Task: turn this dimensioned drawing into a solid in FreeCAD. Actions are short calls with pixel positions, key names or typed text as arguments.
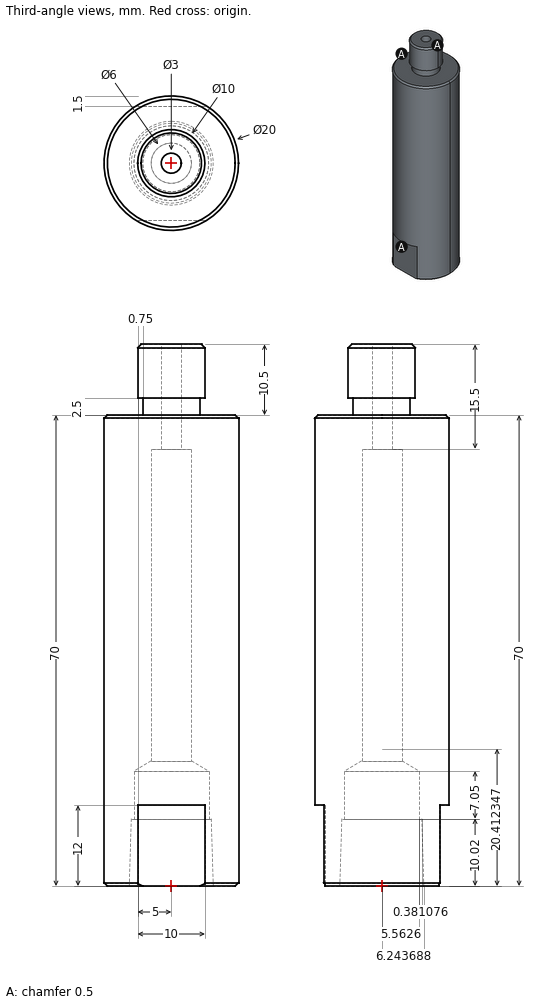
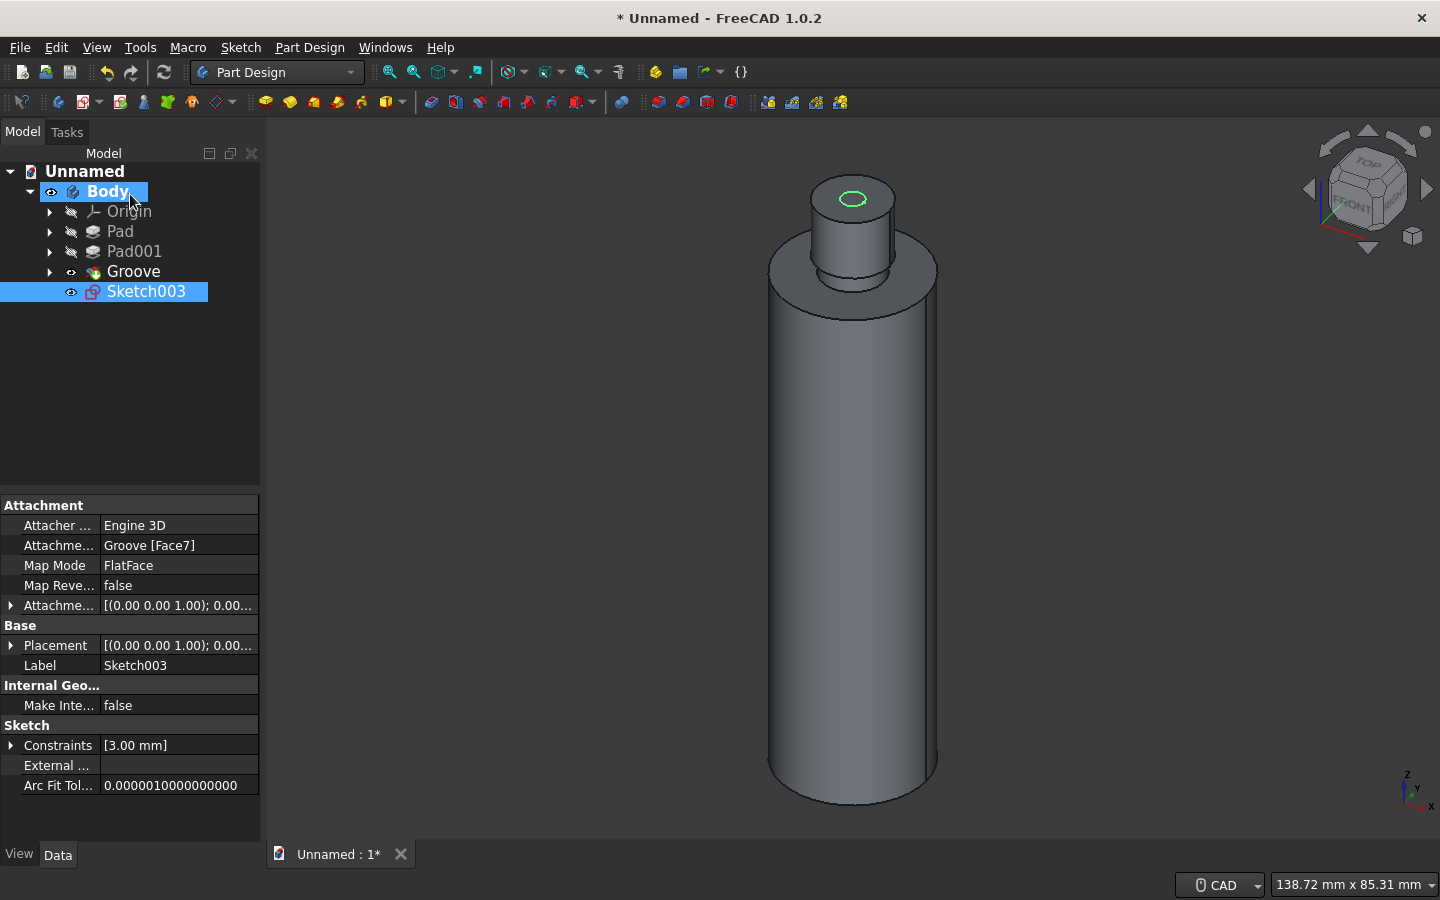
click(432, 102)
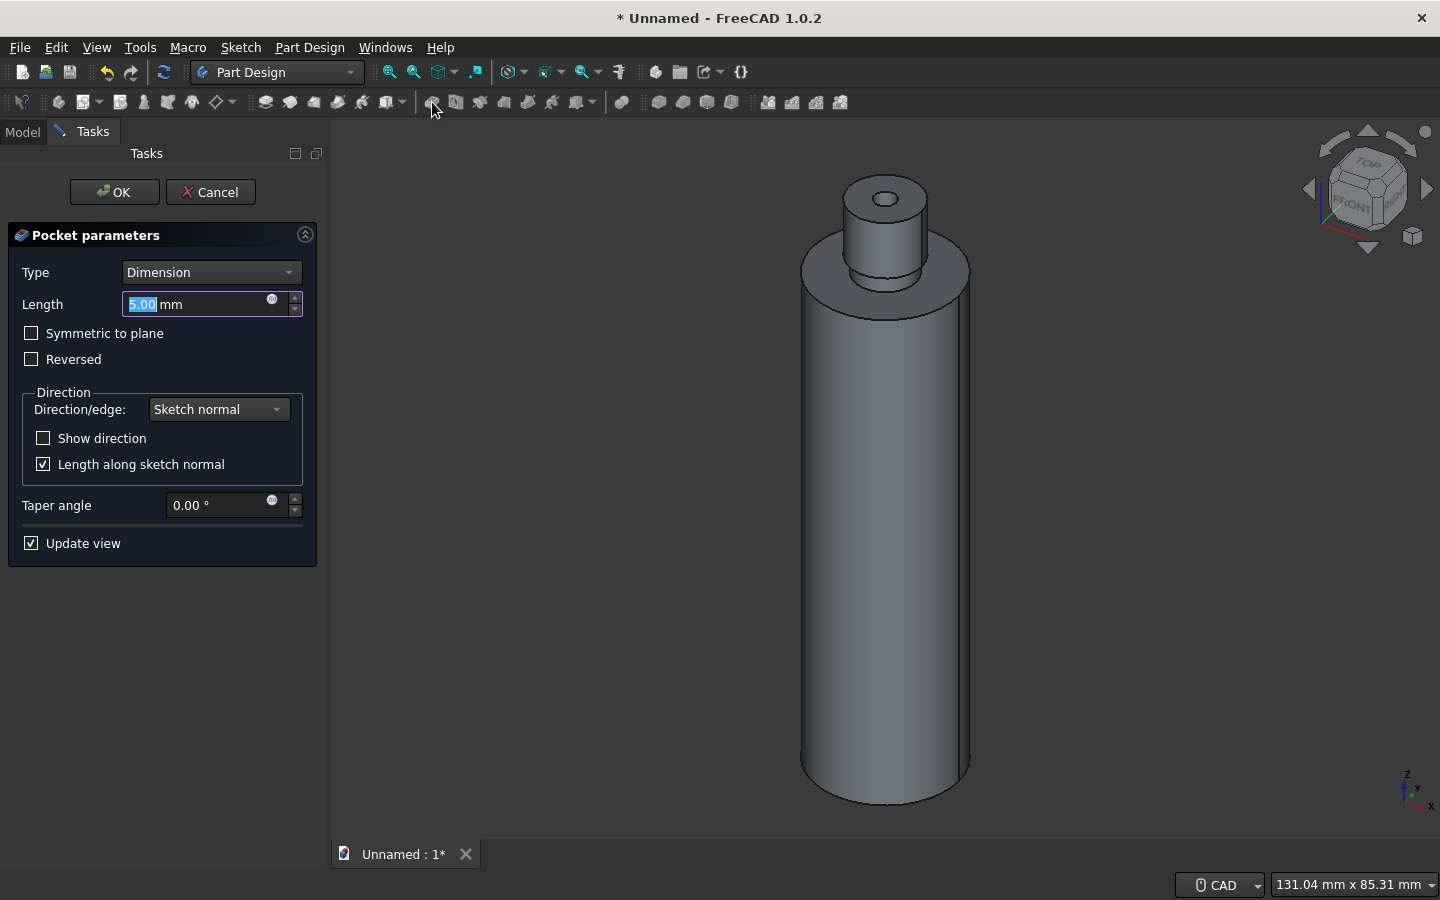
text(15.5)
key(Tab)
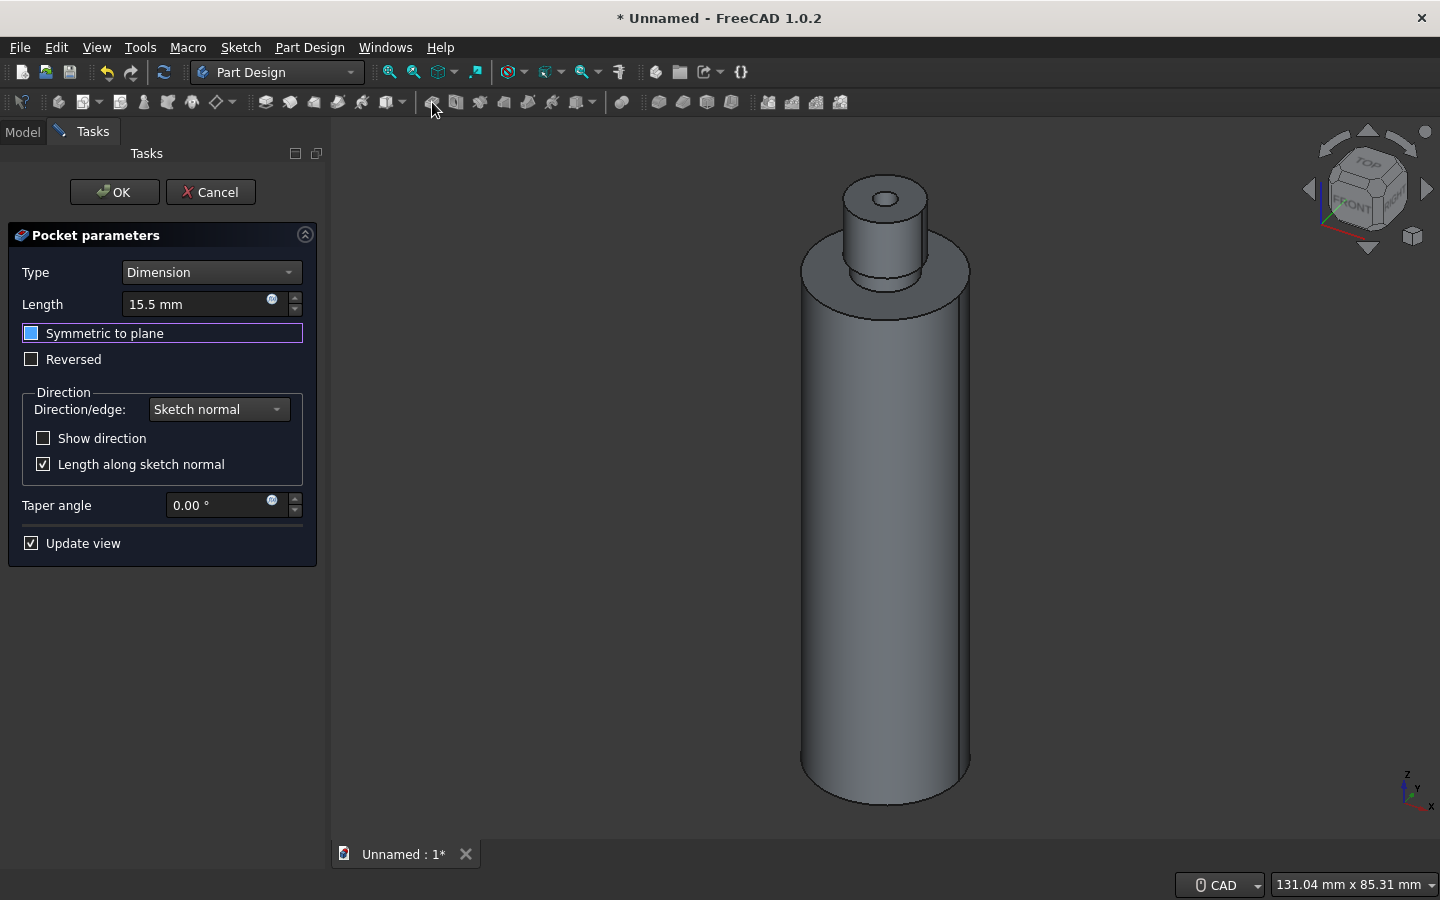
click(115, 192)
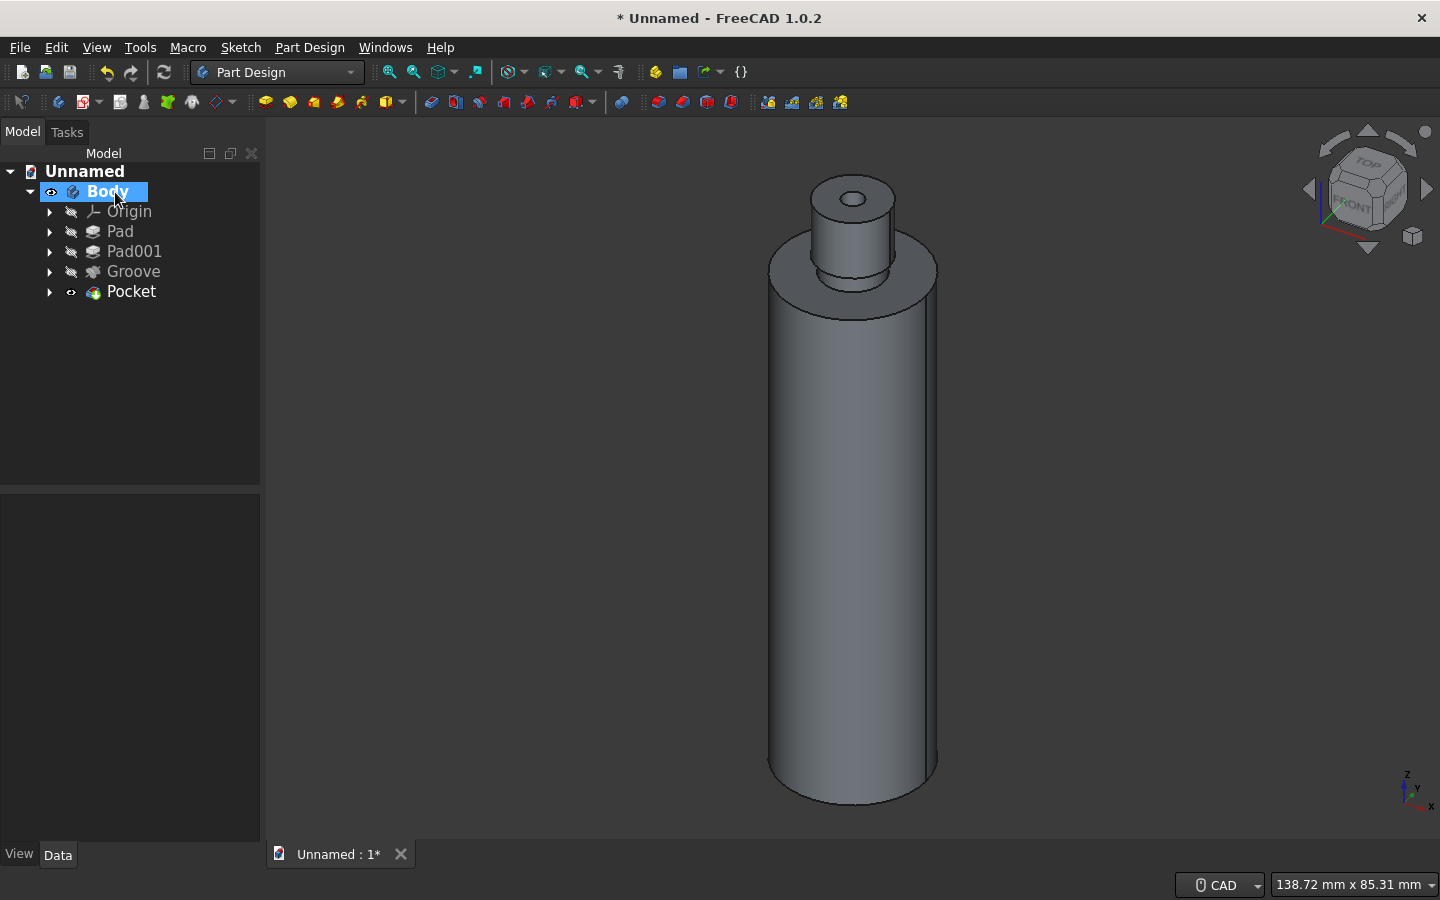
click(84, 102)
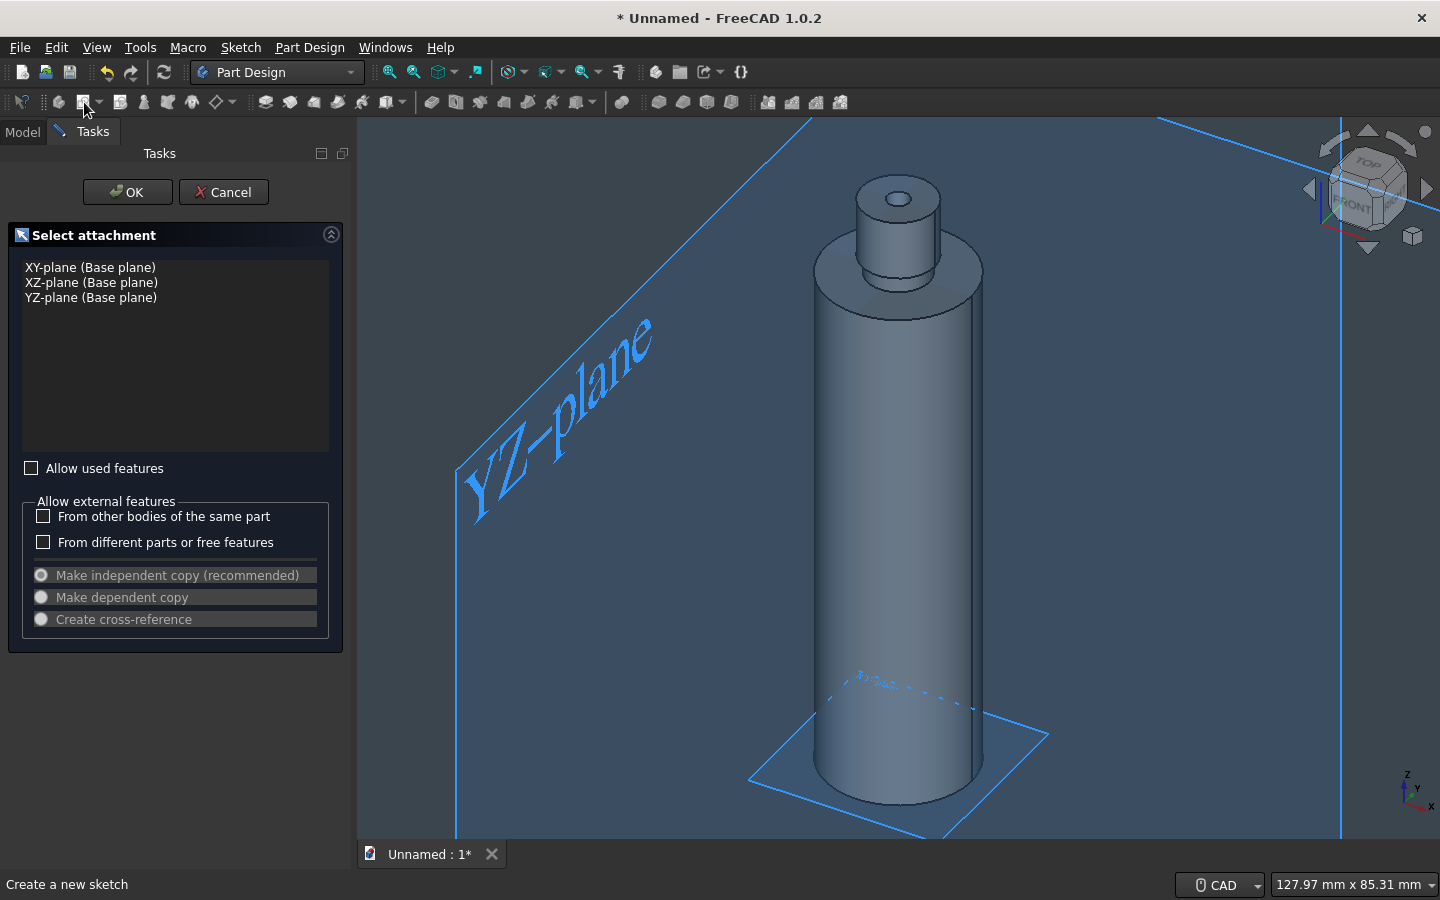
click(82, 298)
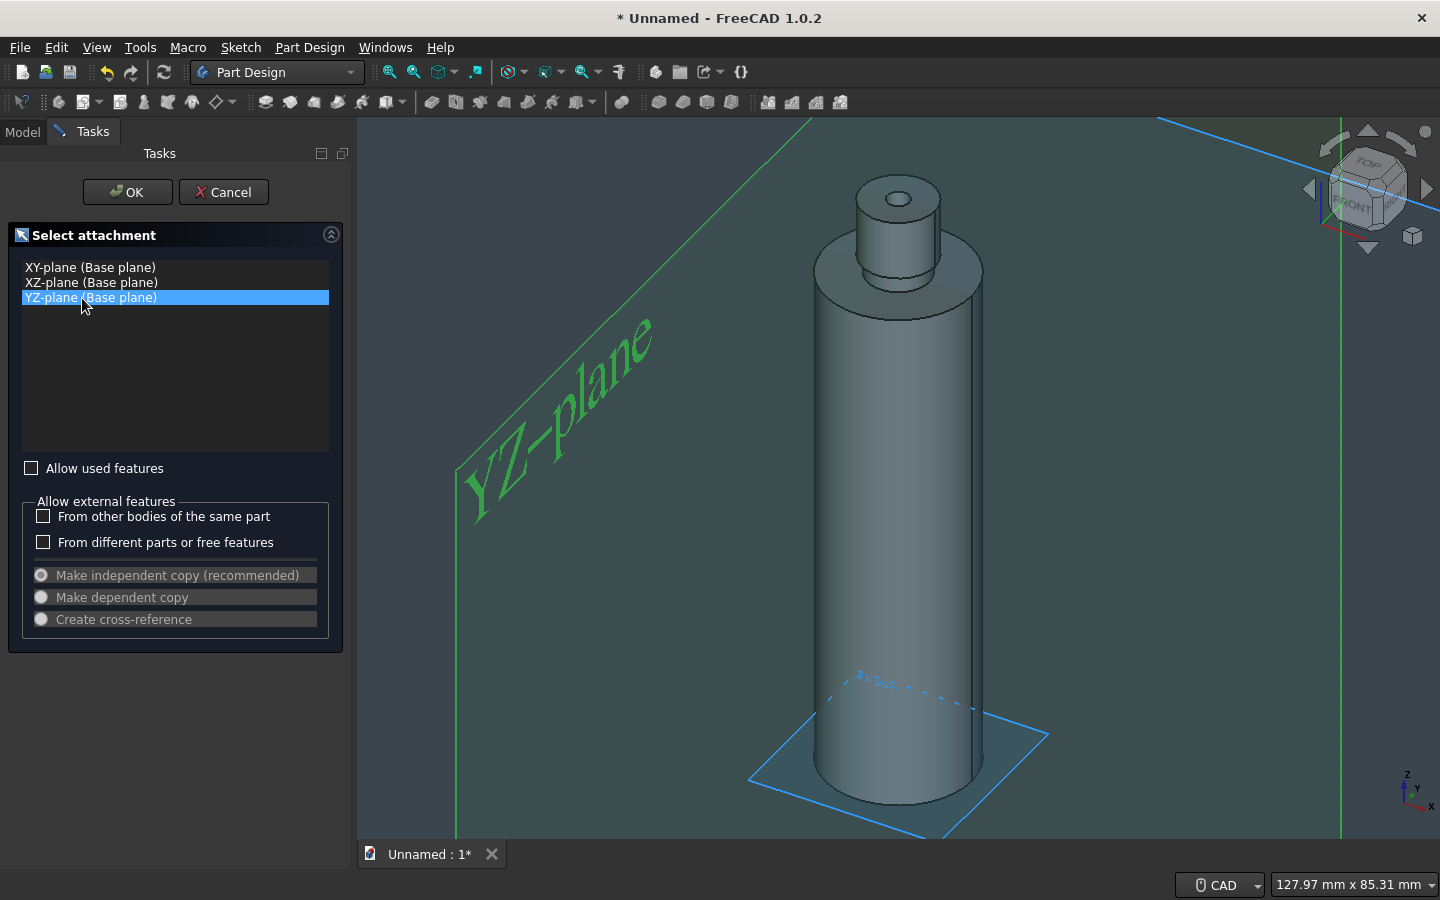
click(128, 192)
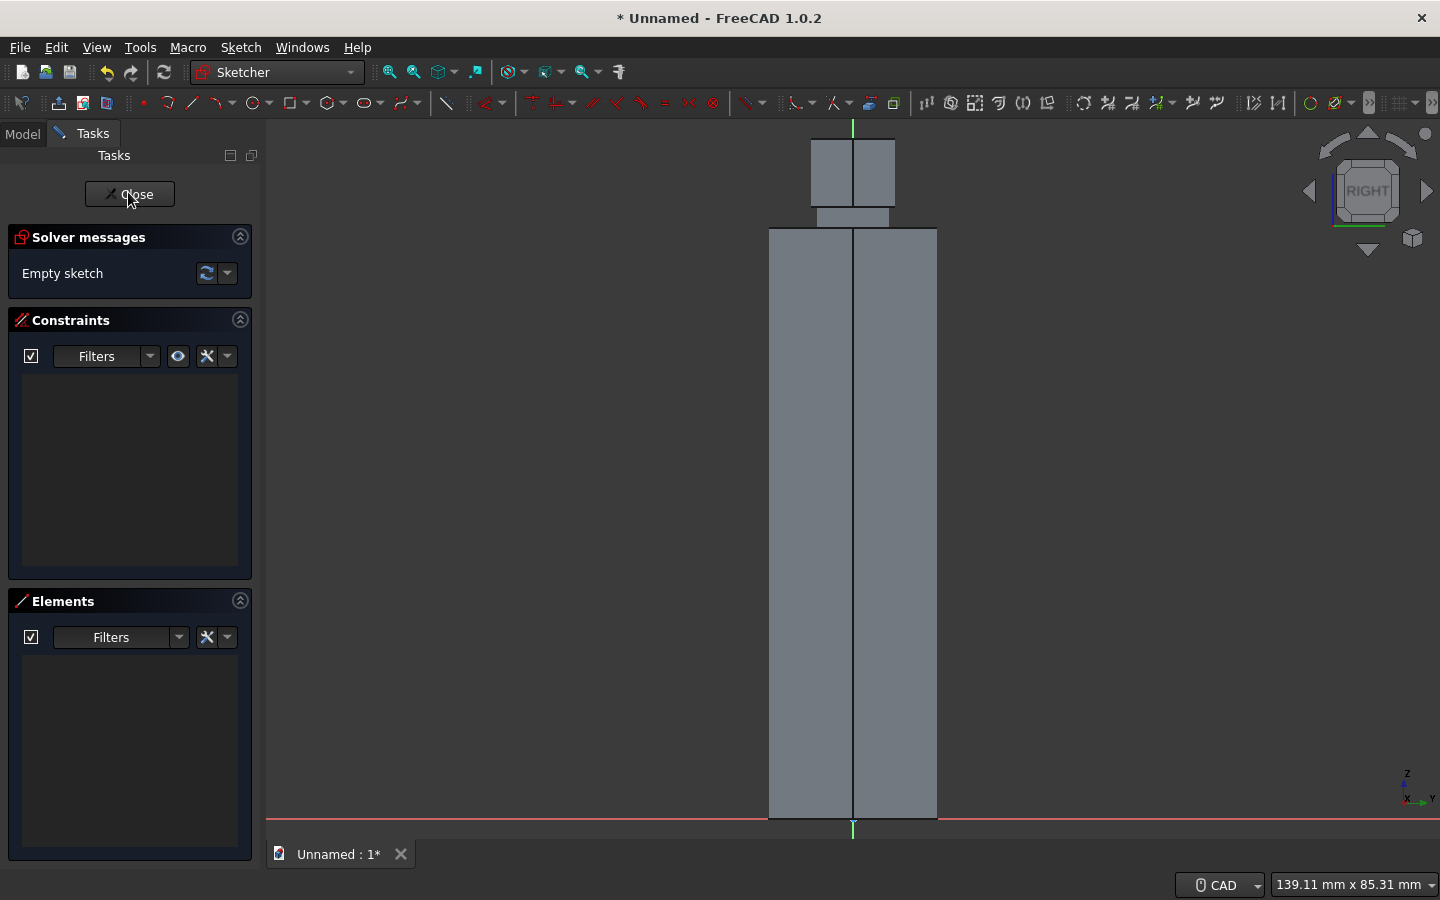
click(108, 104)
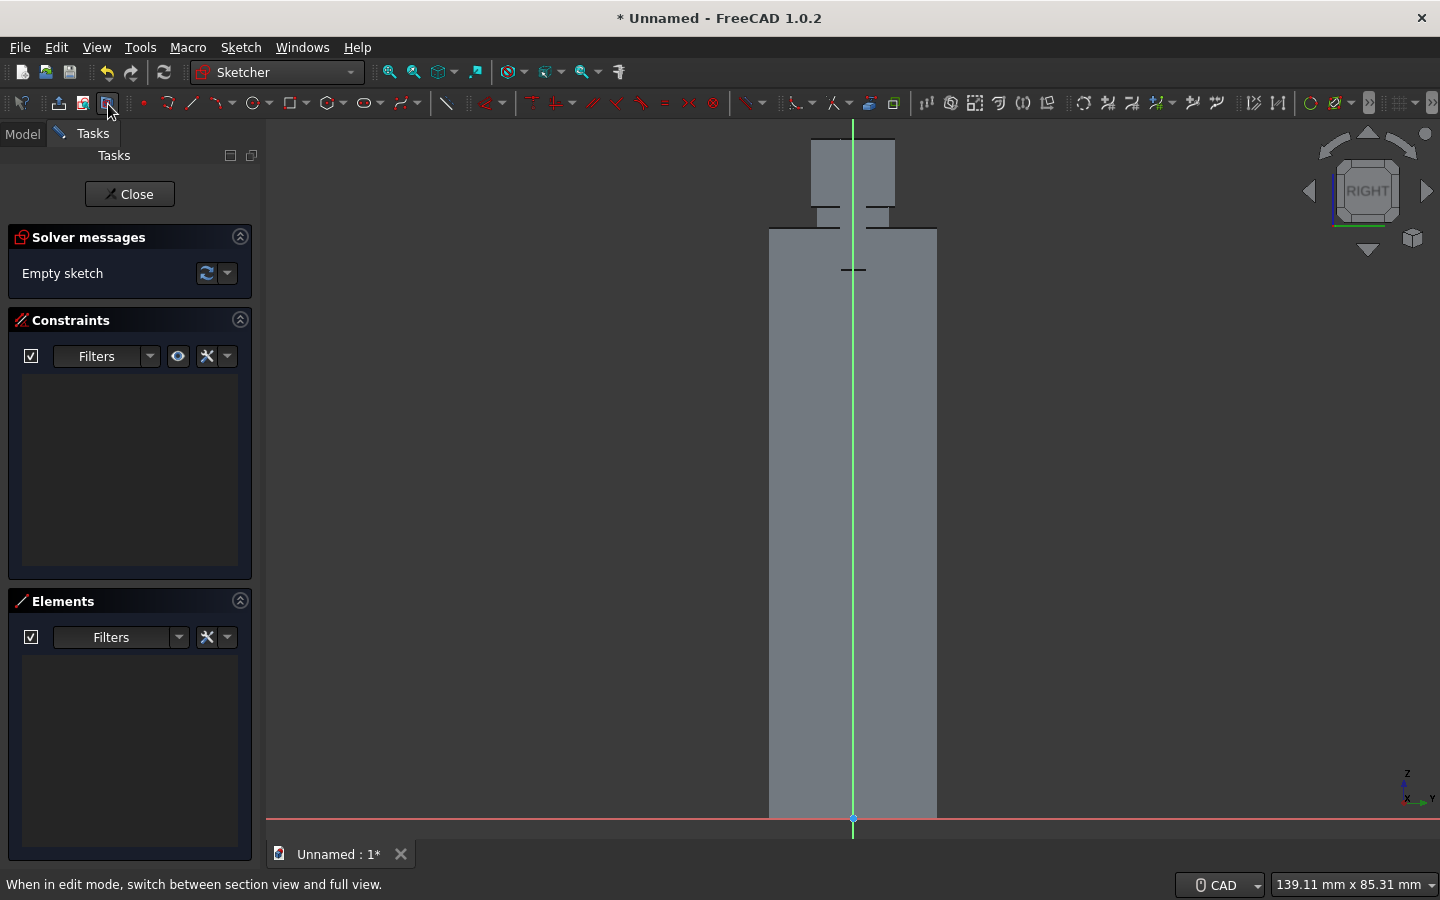
scroll(784, 479, down, 5)